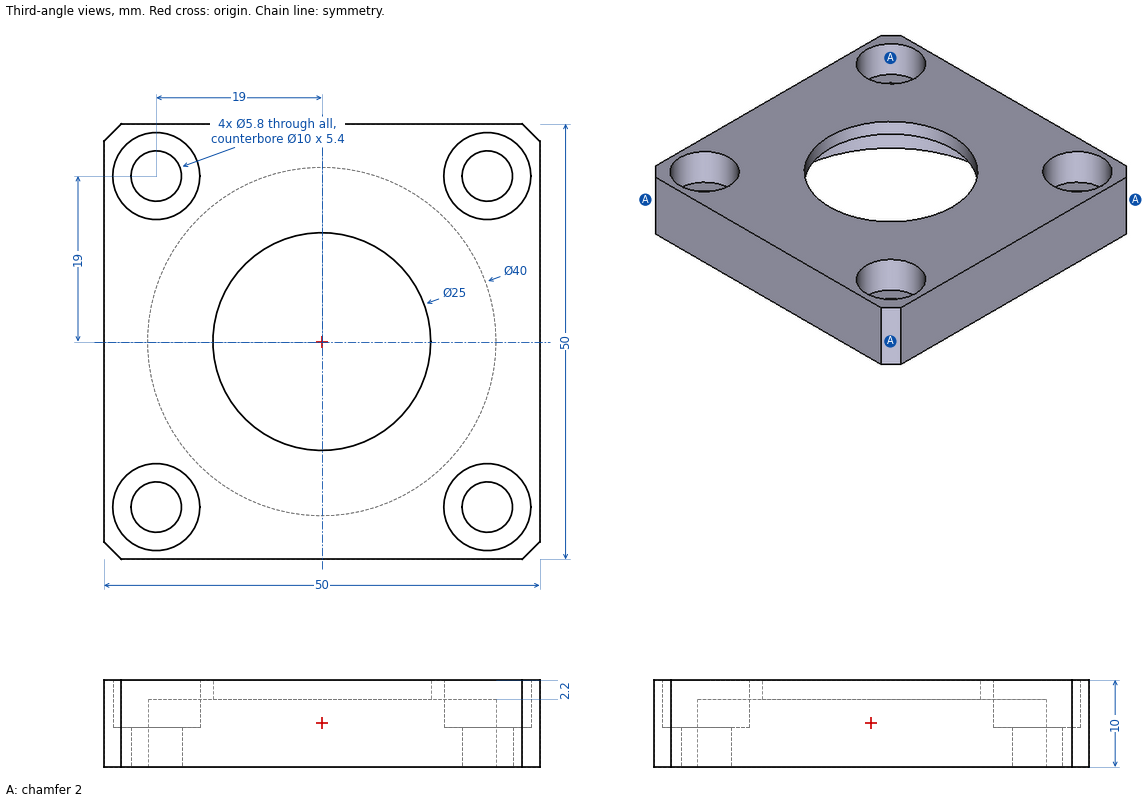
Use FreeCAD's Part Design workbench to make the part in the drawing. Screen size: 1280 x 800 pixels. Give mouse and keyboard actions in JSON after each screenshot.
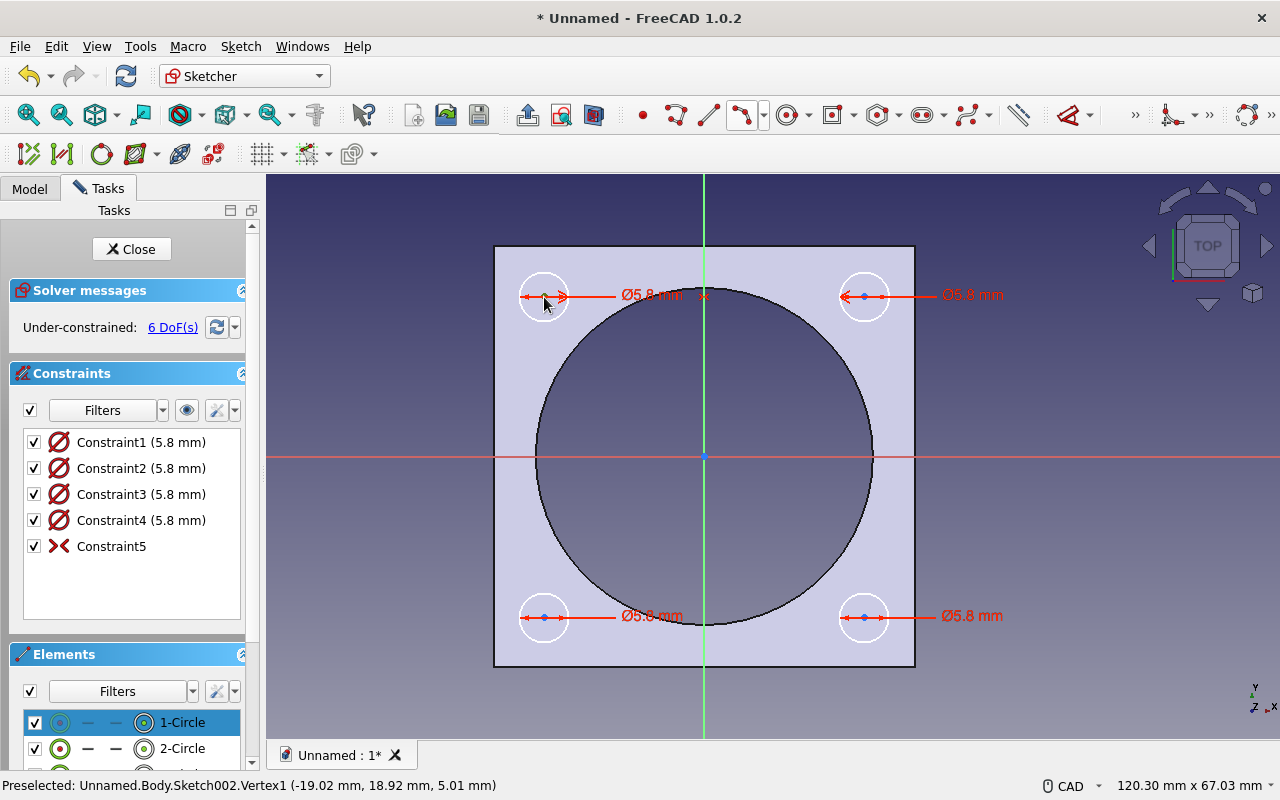
{"action": "left_click", "coordinate": [544, 618]}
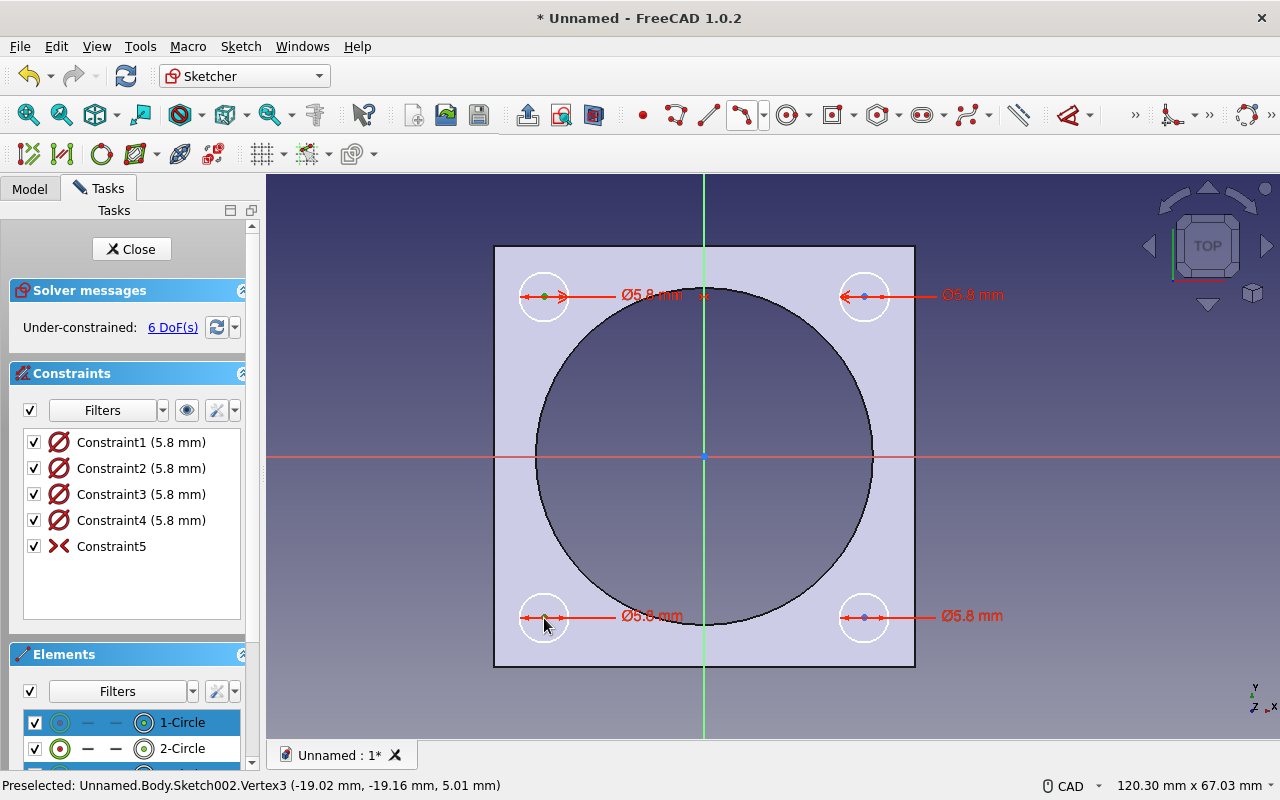
{"action": "left_click", "coordinate": [353, 456]}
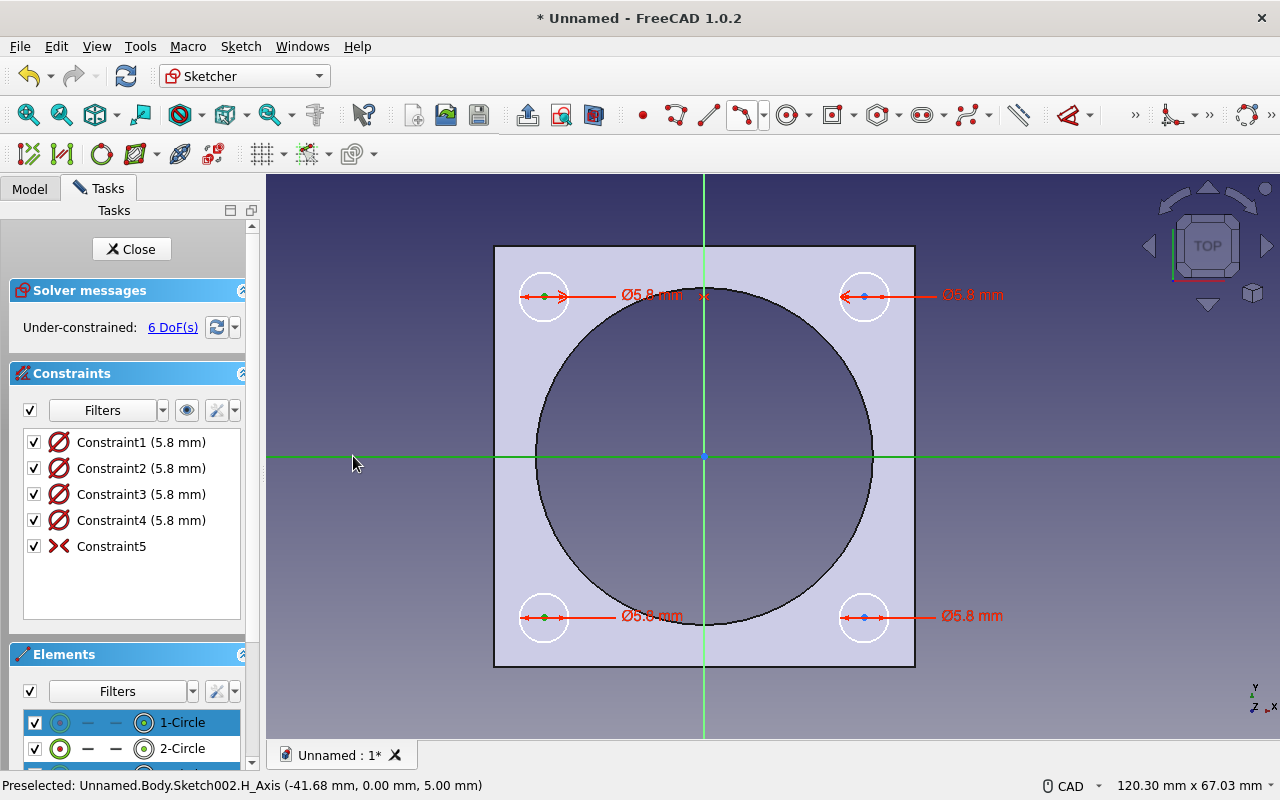
{"action": "key", "text": "s"}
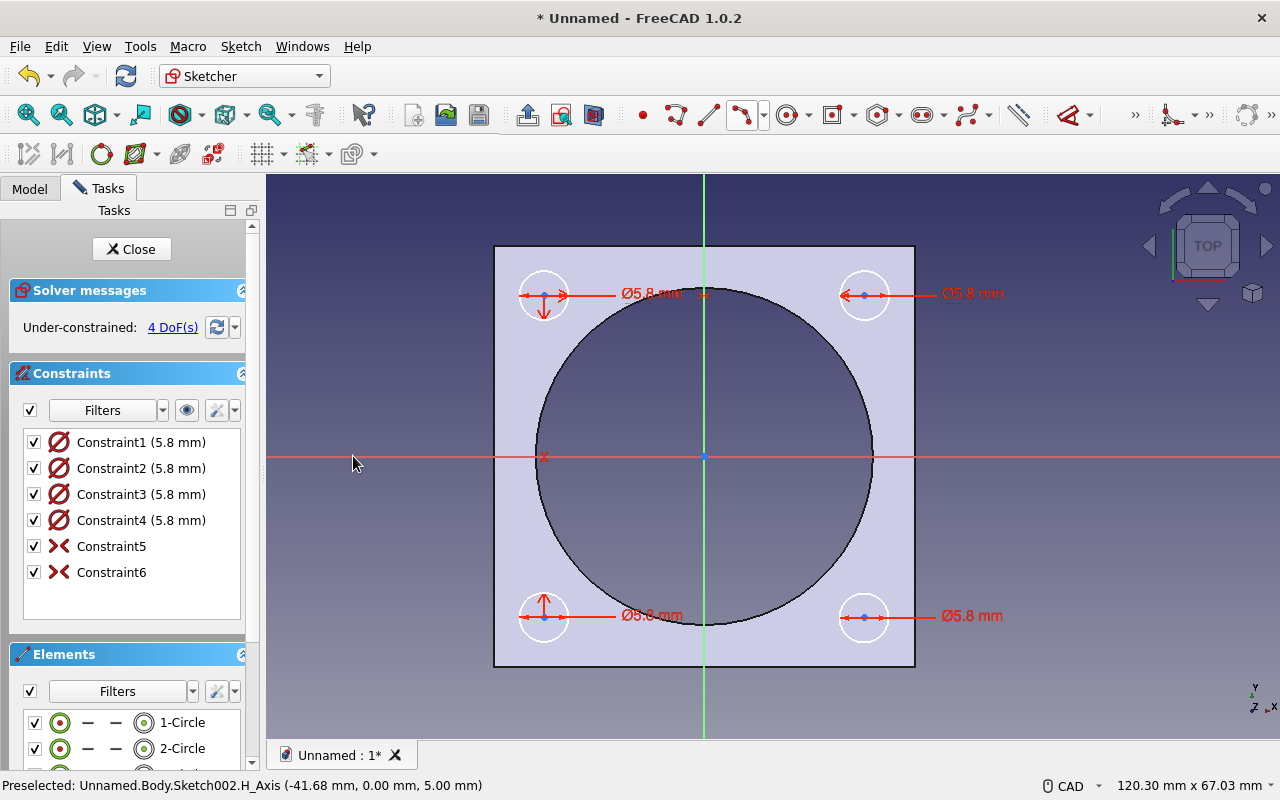
{"action": "left_click", "coordinate": [865, 296]}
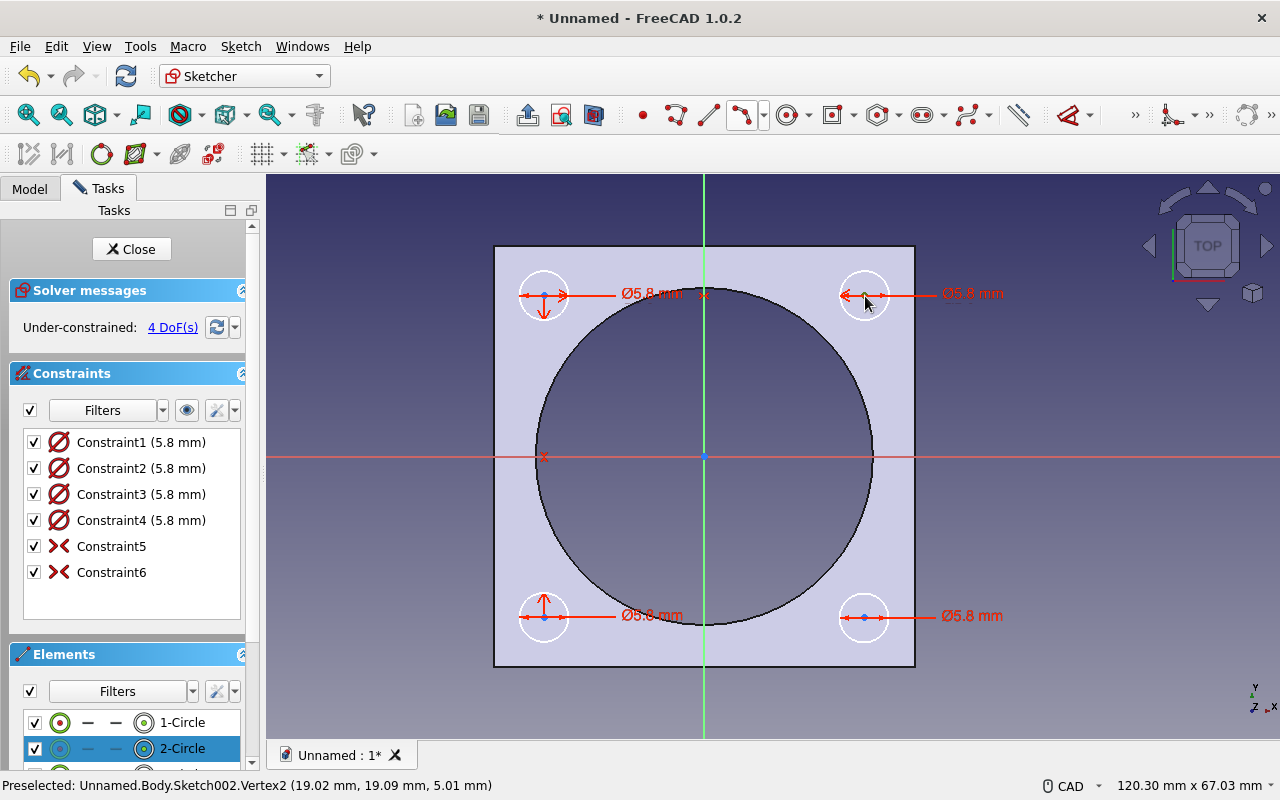
{"action": "left_click", "coordinate": [864, 618]}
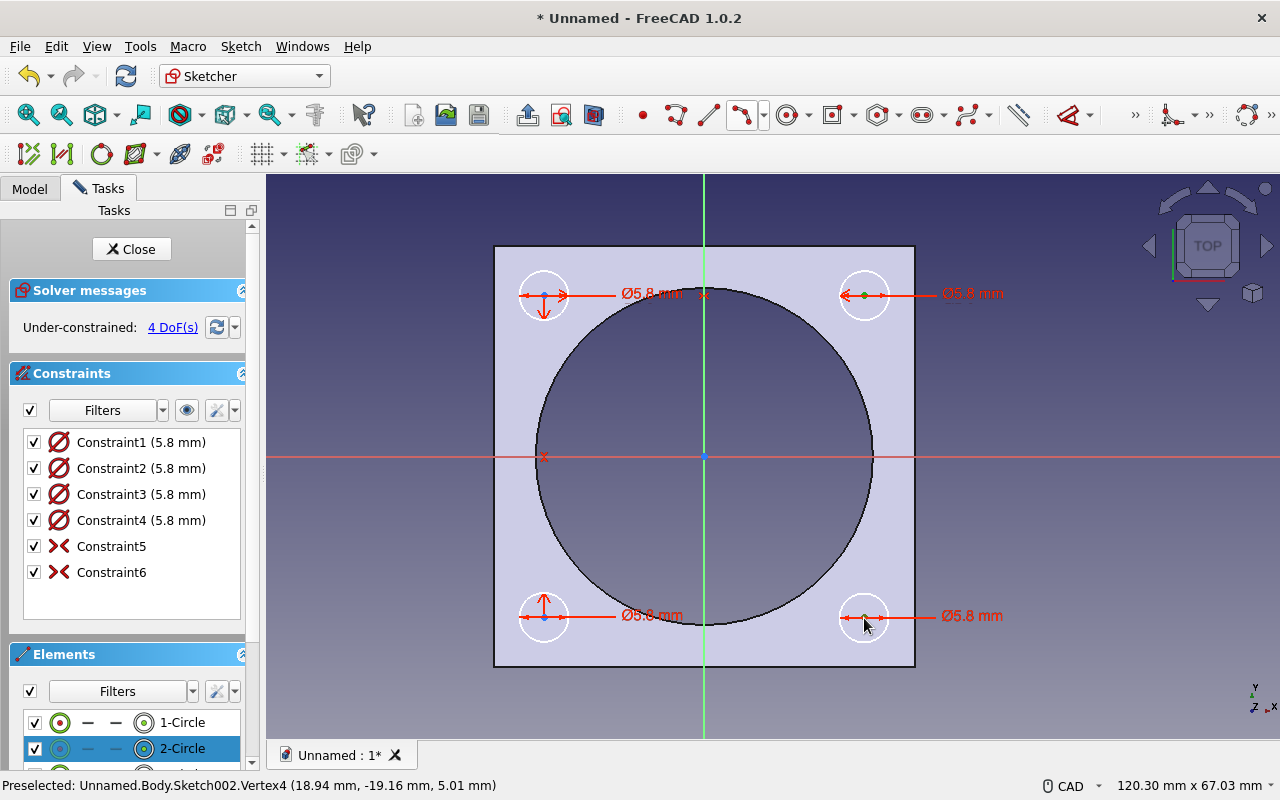
{"action": "left_click", "coordinate": [353, 456]}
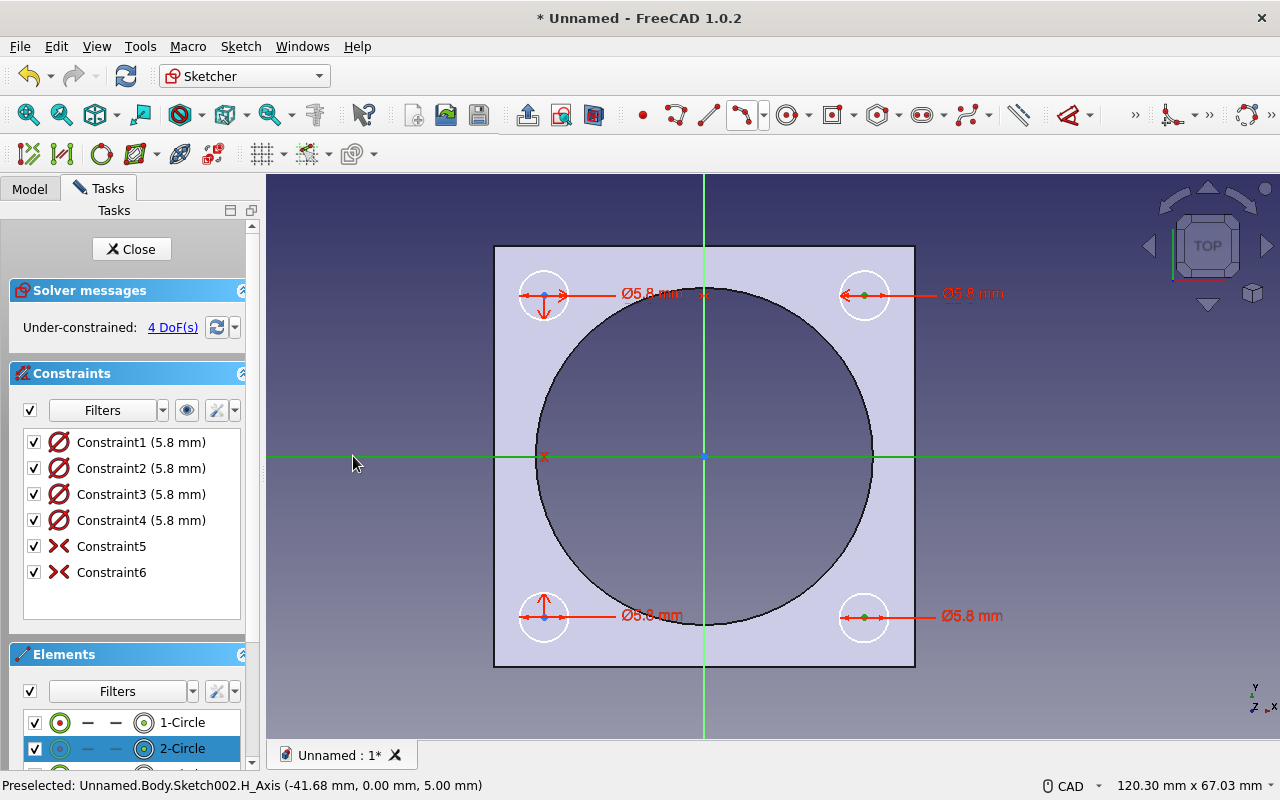
{"action": "key", "text": "s"}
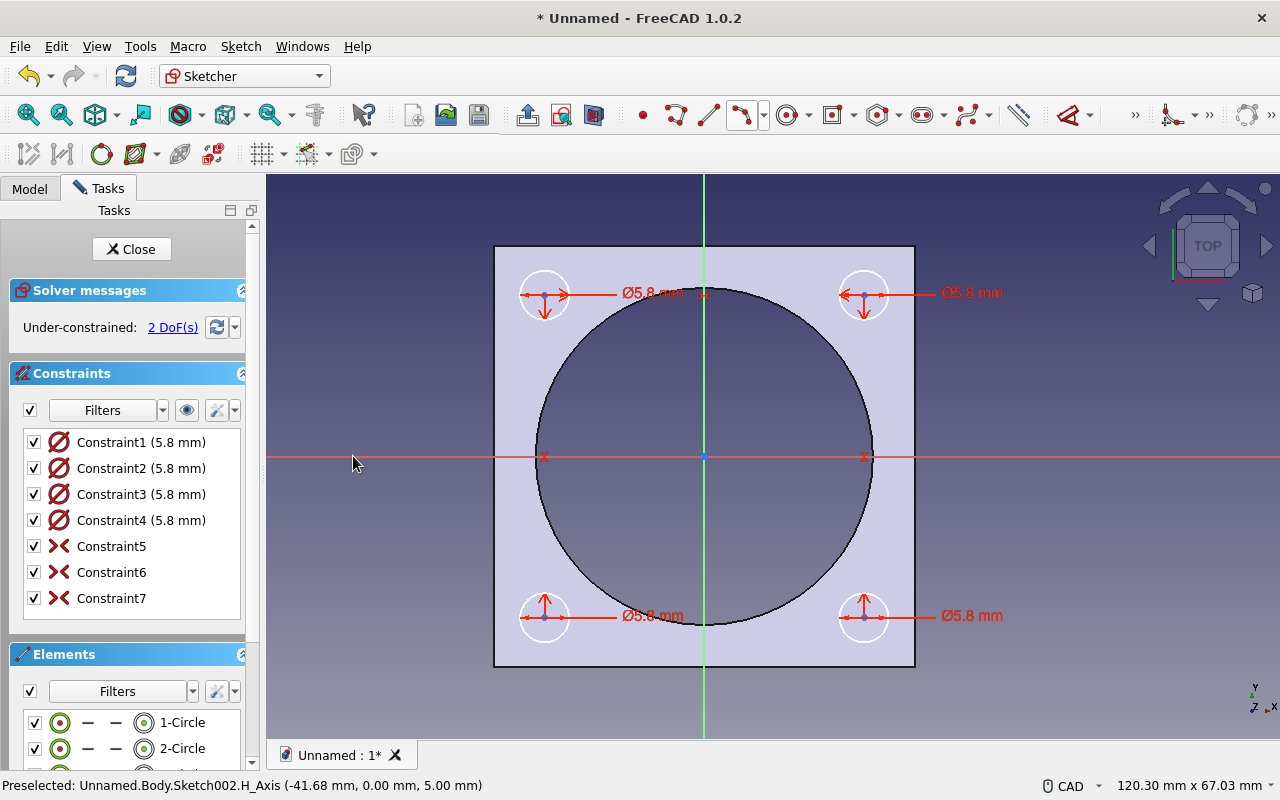
{"action": "left_click", "coordinate": [1068, 116]}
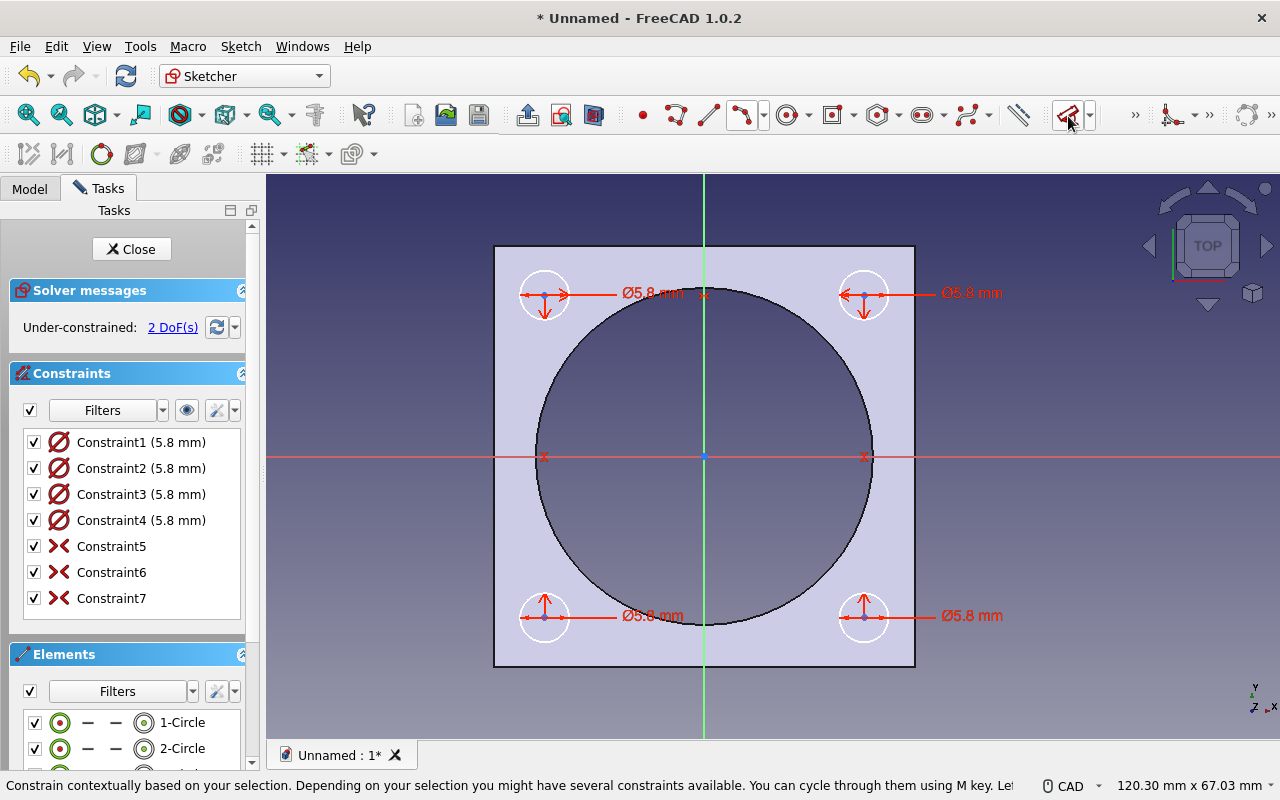
{"action": "left_click", "coordinate": [545, 295]}
{"action": "left_click", "coordinate": [624, 261]}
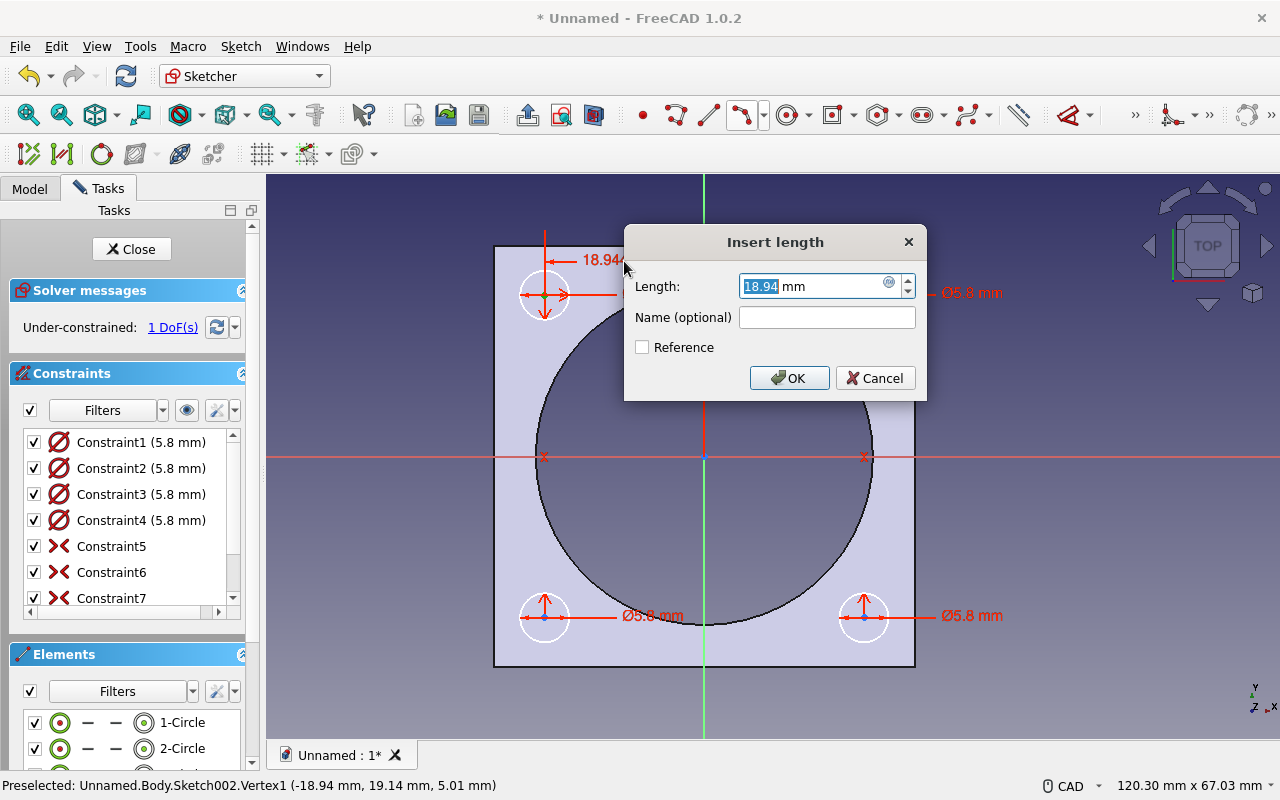
{"action": "type", "text": "19"}
{"action": "key", "text": "Return"}